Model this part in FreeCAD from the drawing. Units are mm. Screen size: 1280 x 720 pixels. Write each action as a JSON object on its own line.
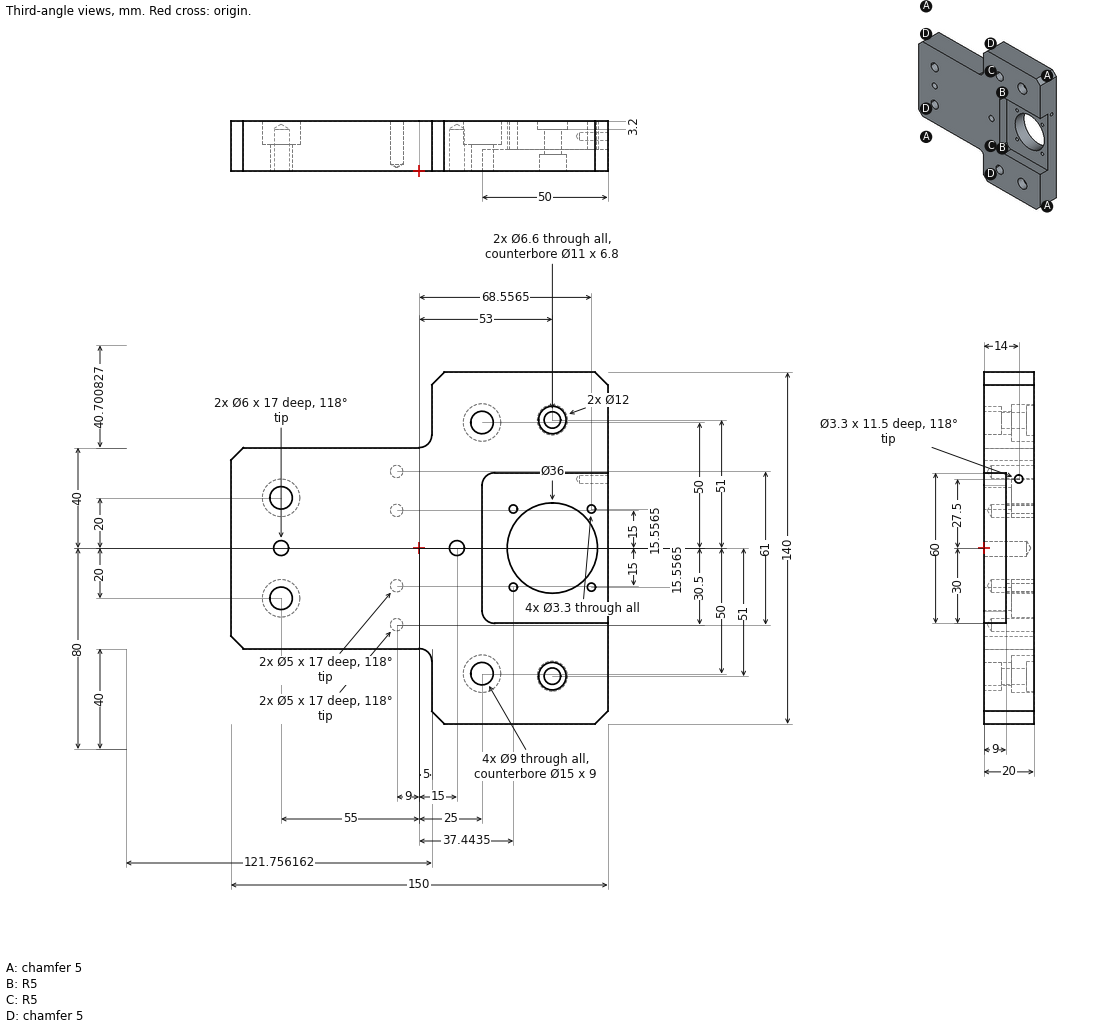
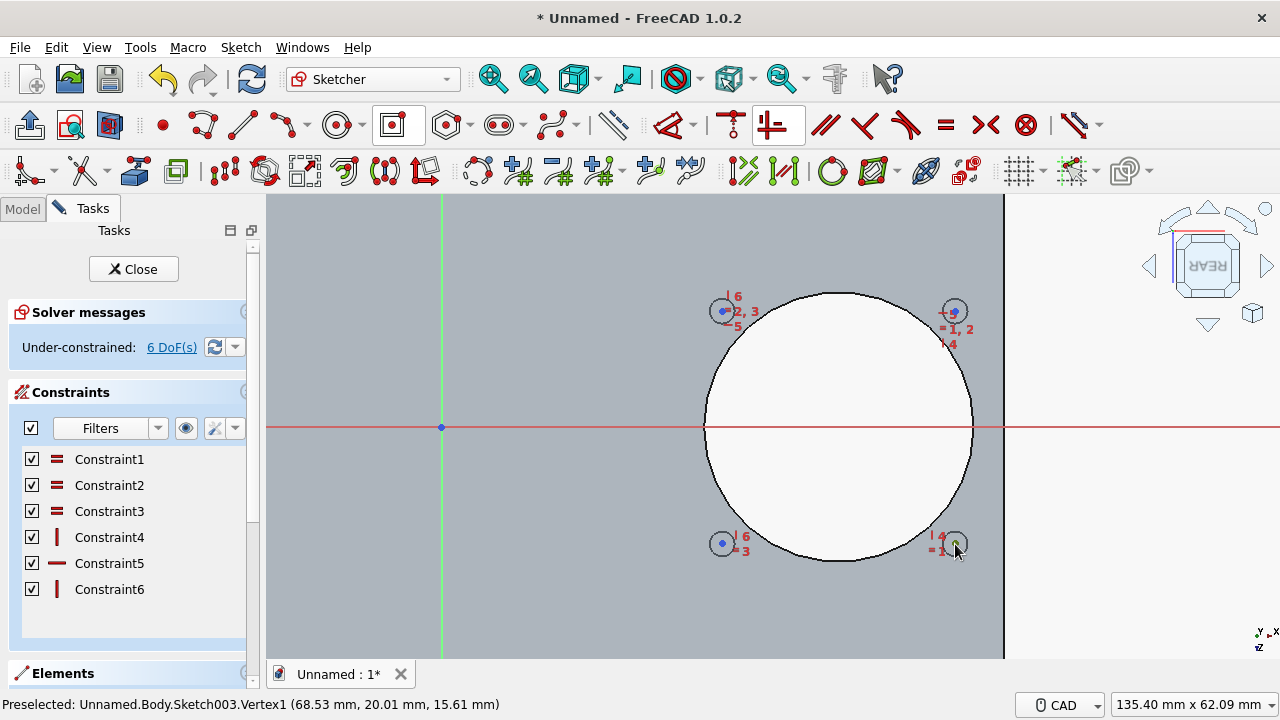
{"action": "left_click", "coordinate": [722, 544]}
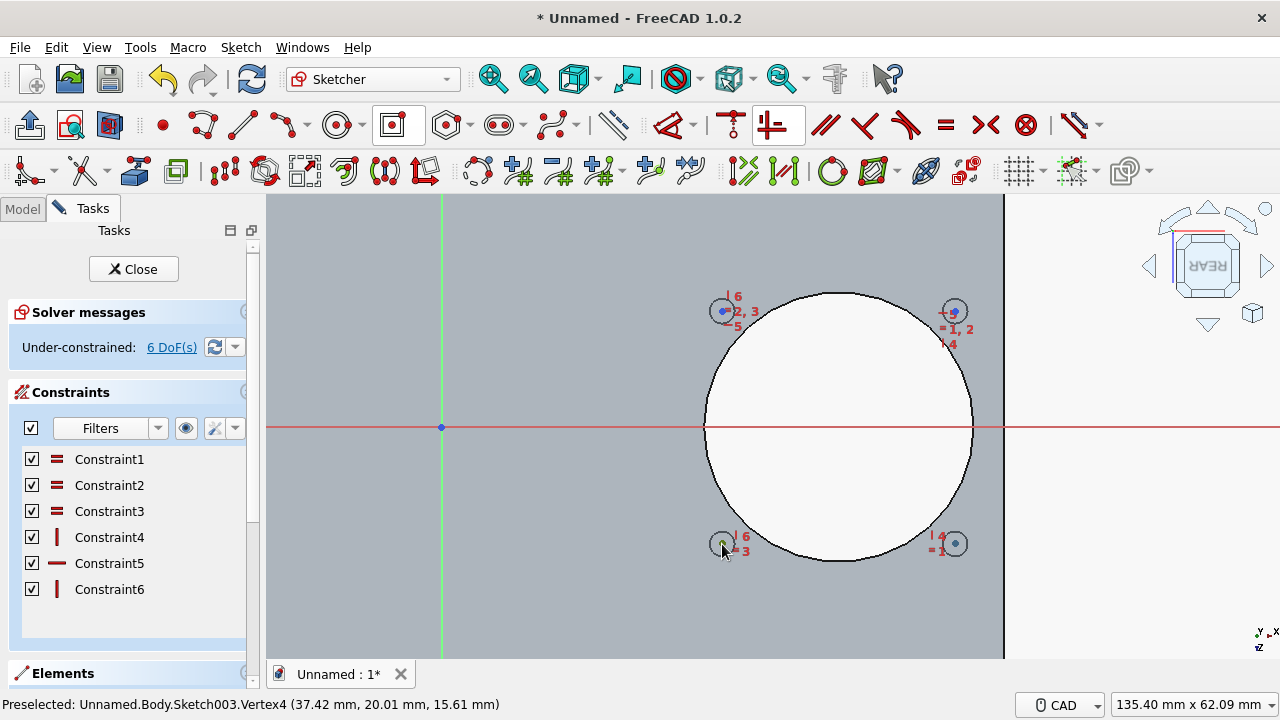
{"action": "left_click", "coordinate": [800, 126]}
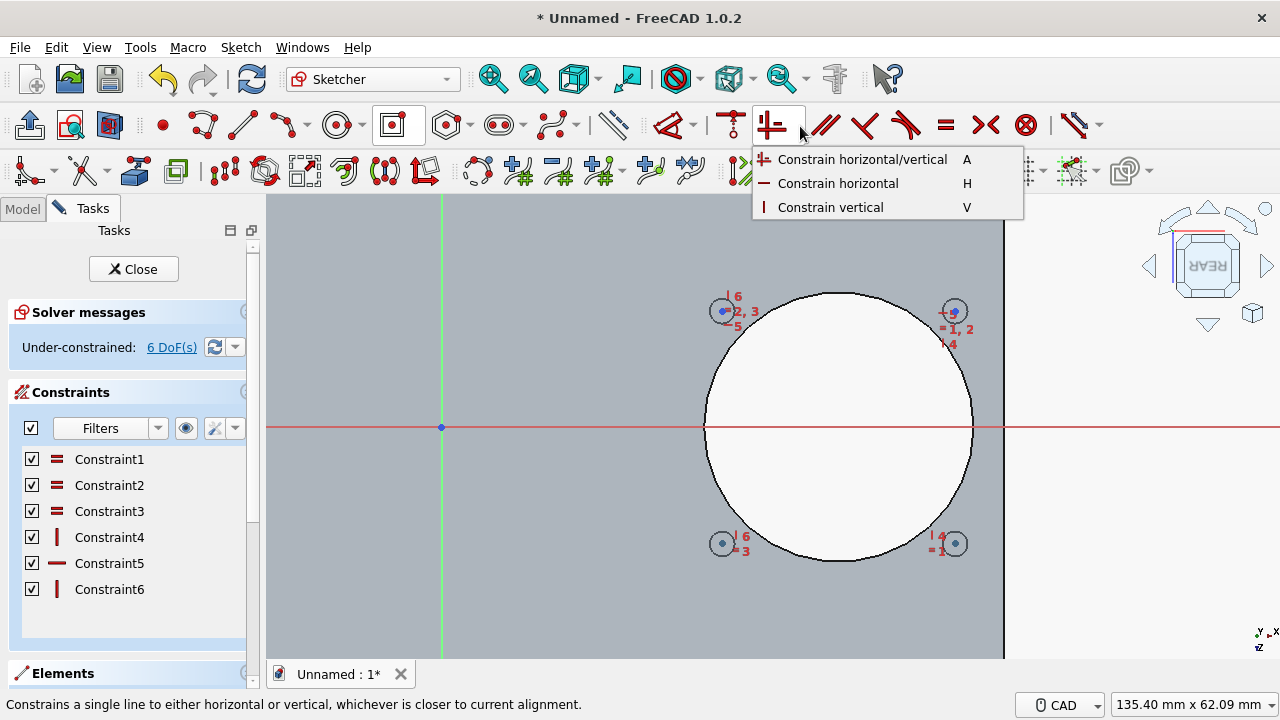
{"action": "left_click", "coordinate": [888, 183]}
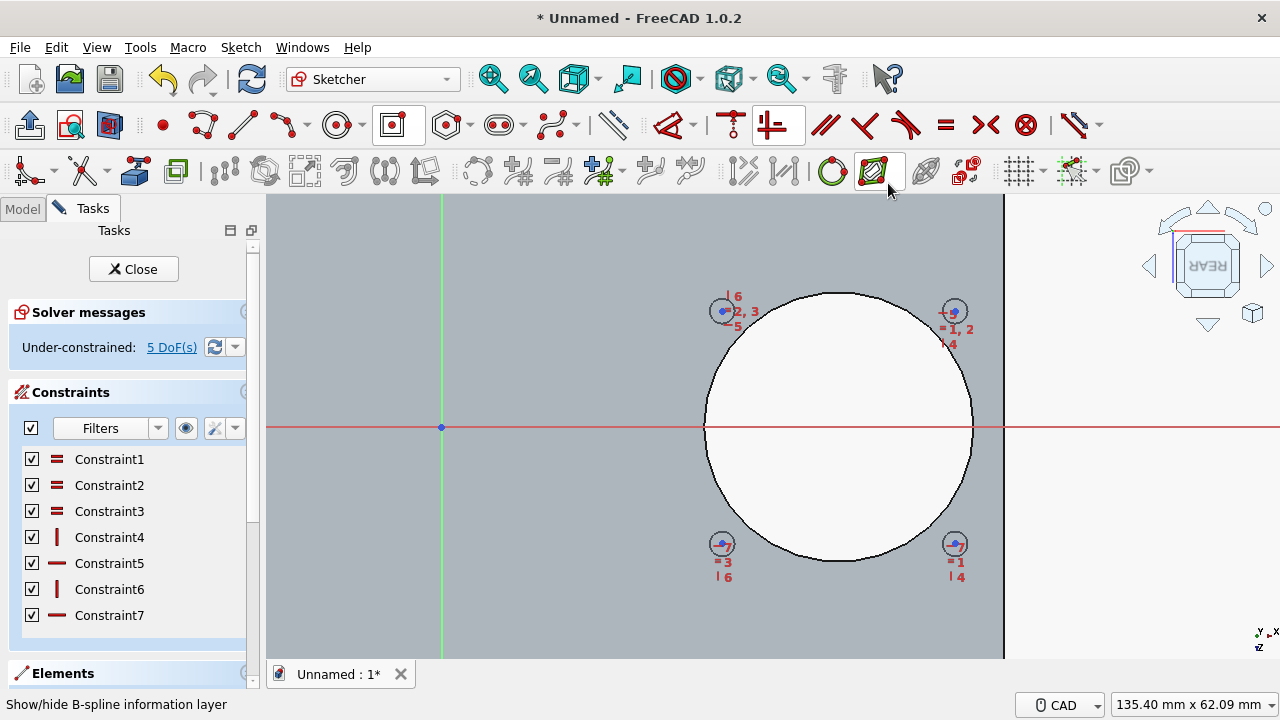
{"action": "left_click", "coordinate": [668, 126]}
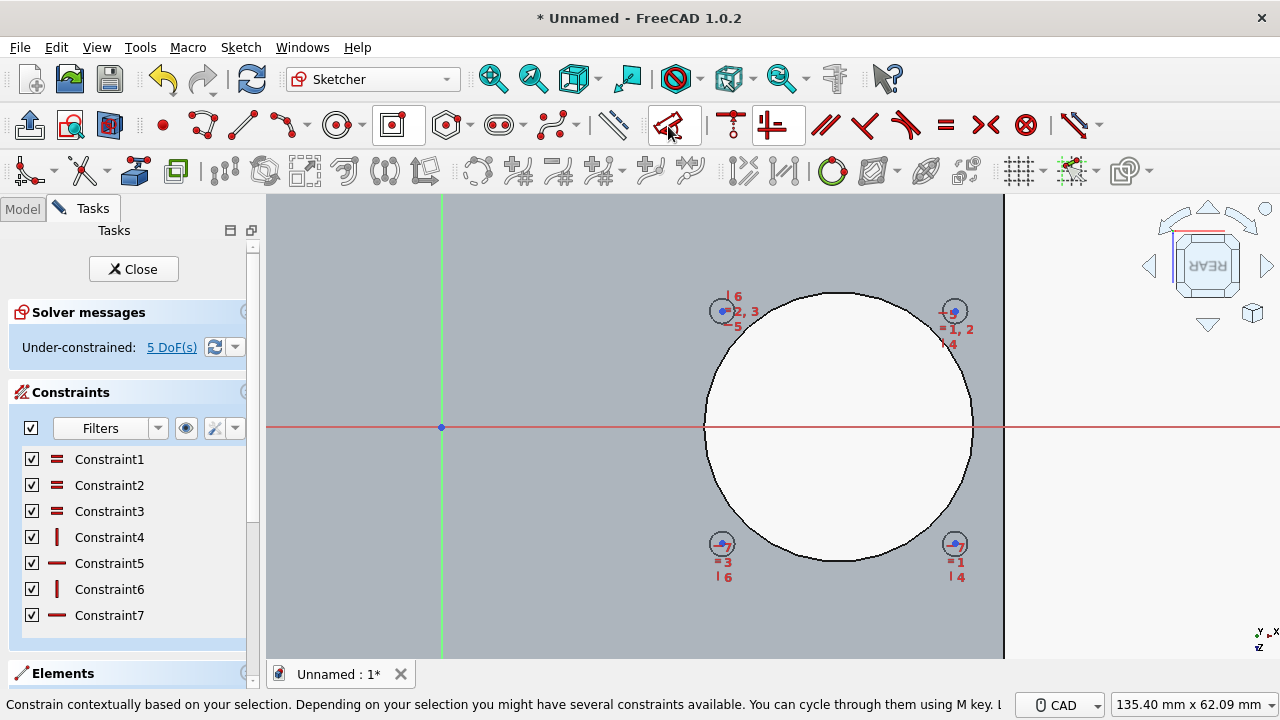
{"action": "scroll", "coordinate": [964, 535], "scroll_direction": "up", "scroll_amount": 3}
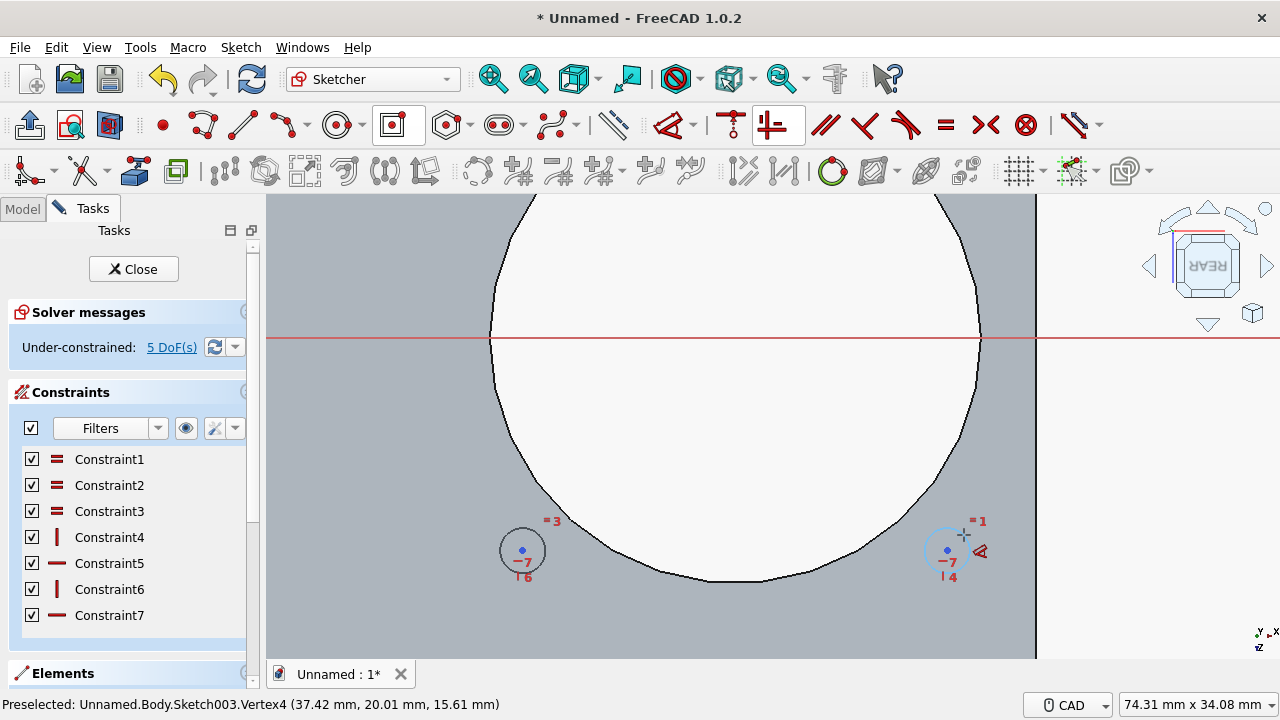
{"action": "left_click", "coordinate": [963, 535]}
{"action": "left_click", "coordinate": [986, 512]}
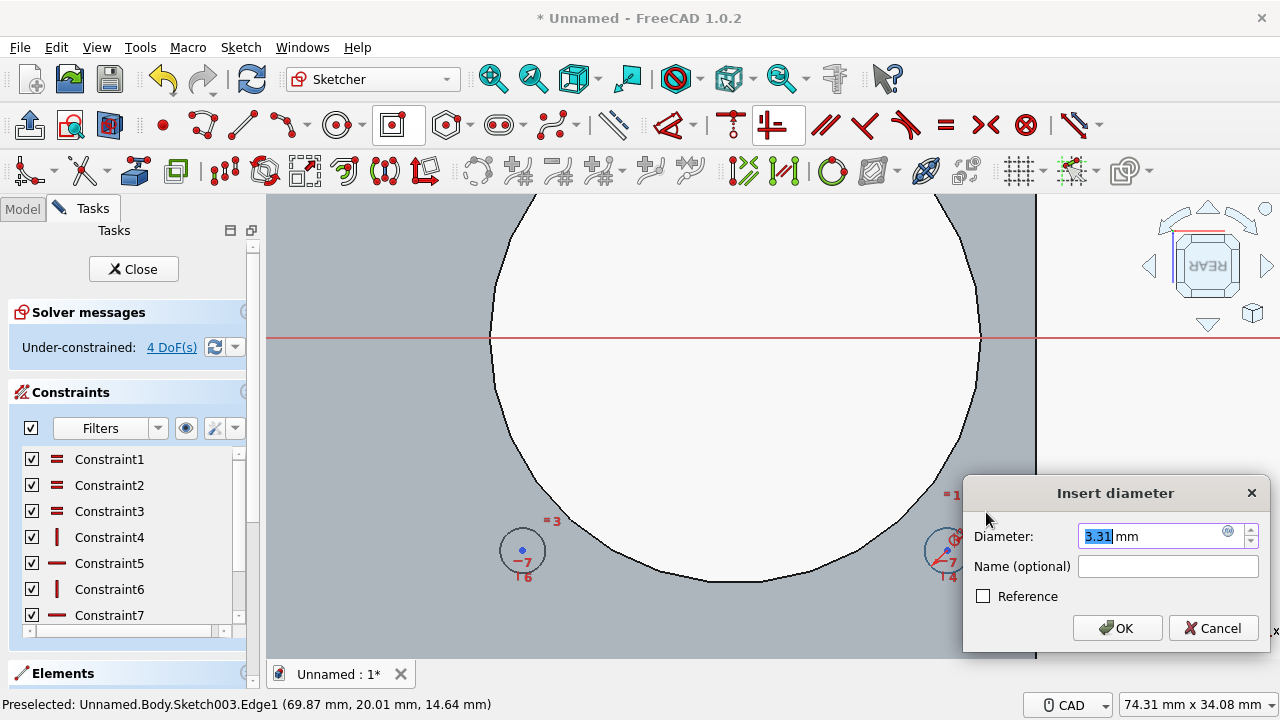
{"action": "type", "text": "3.3"}
{"action": "key", "text": "Return"}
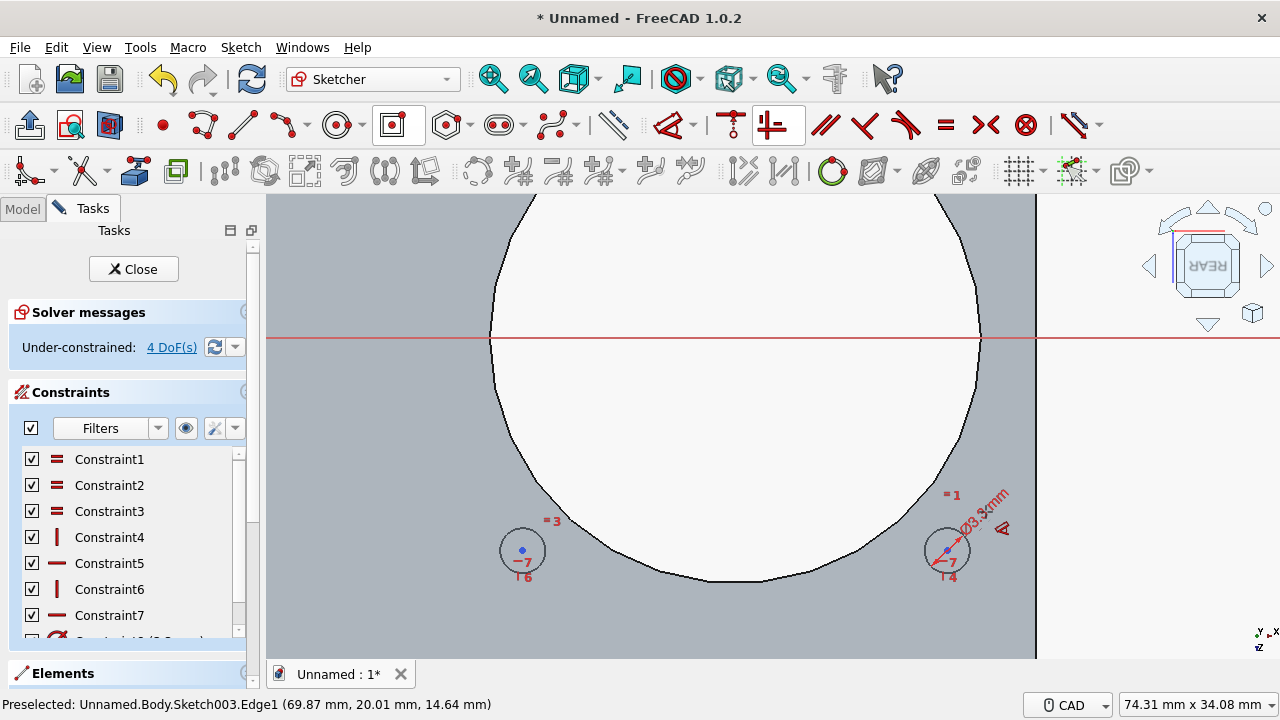
{"action": "left_click", "coordinate": [947, 551]}
{"action": "left_click", "coordinate": [621, 585]}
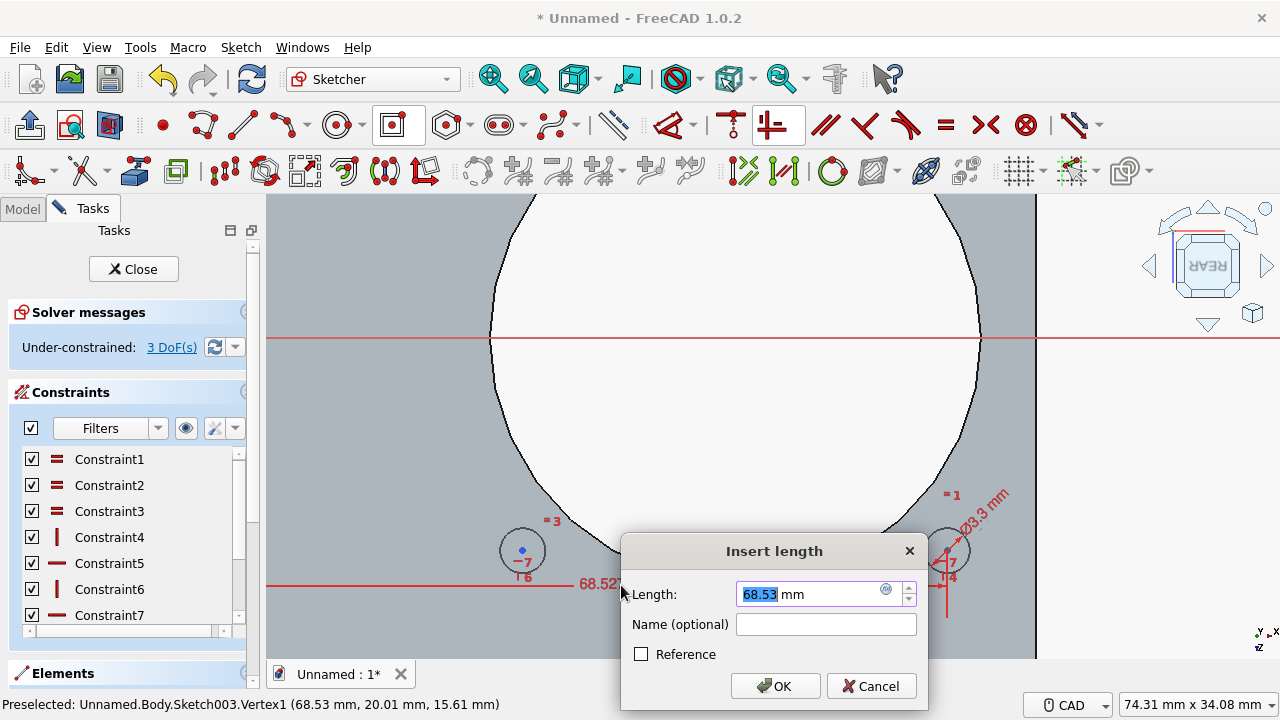
{"action": "type", "text": "68.5565"}
{"action": "key", "text": "Return"}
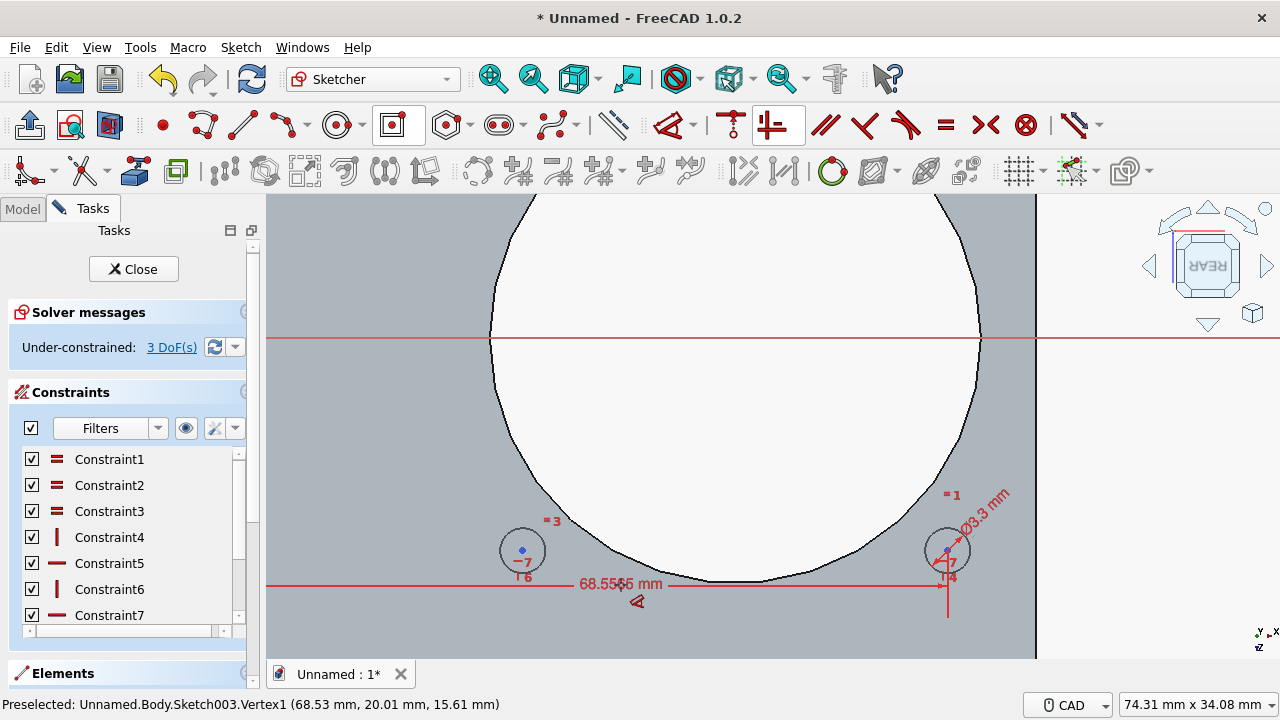
{"action": "left_click", "coordinate": [948, 551]}
{"action": "left_click", "coordinate": [982, 444]}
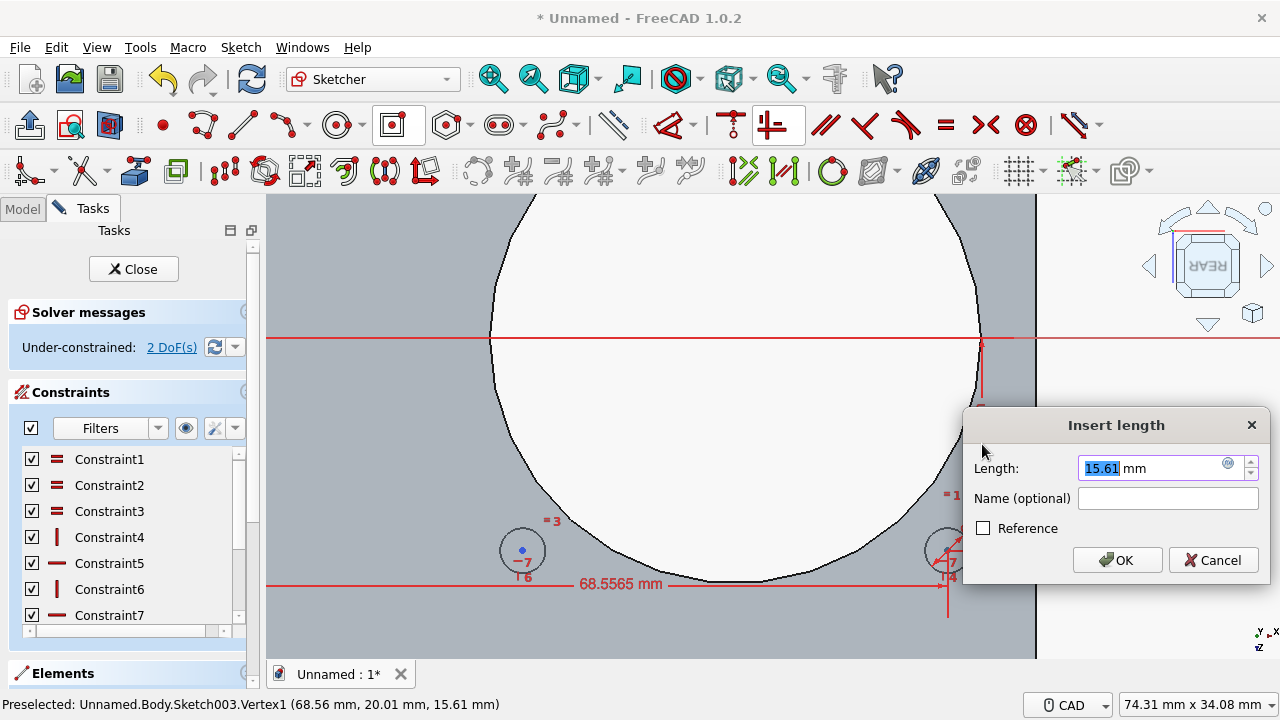
{"action": "type", "text": "15.5565"}
{"action": "key", "text": "Return"}